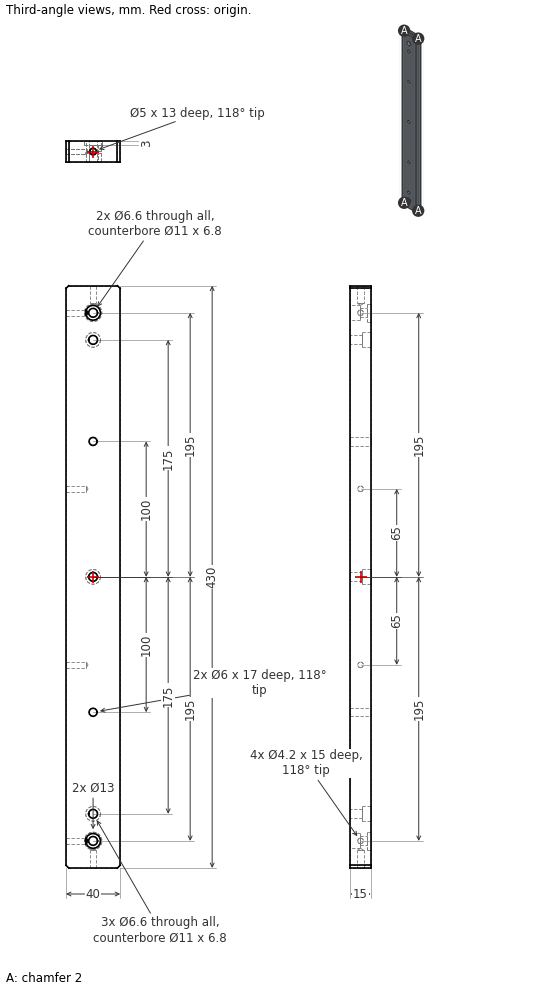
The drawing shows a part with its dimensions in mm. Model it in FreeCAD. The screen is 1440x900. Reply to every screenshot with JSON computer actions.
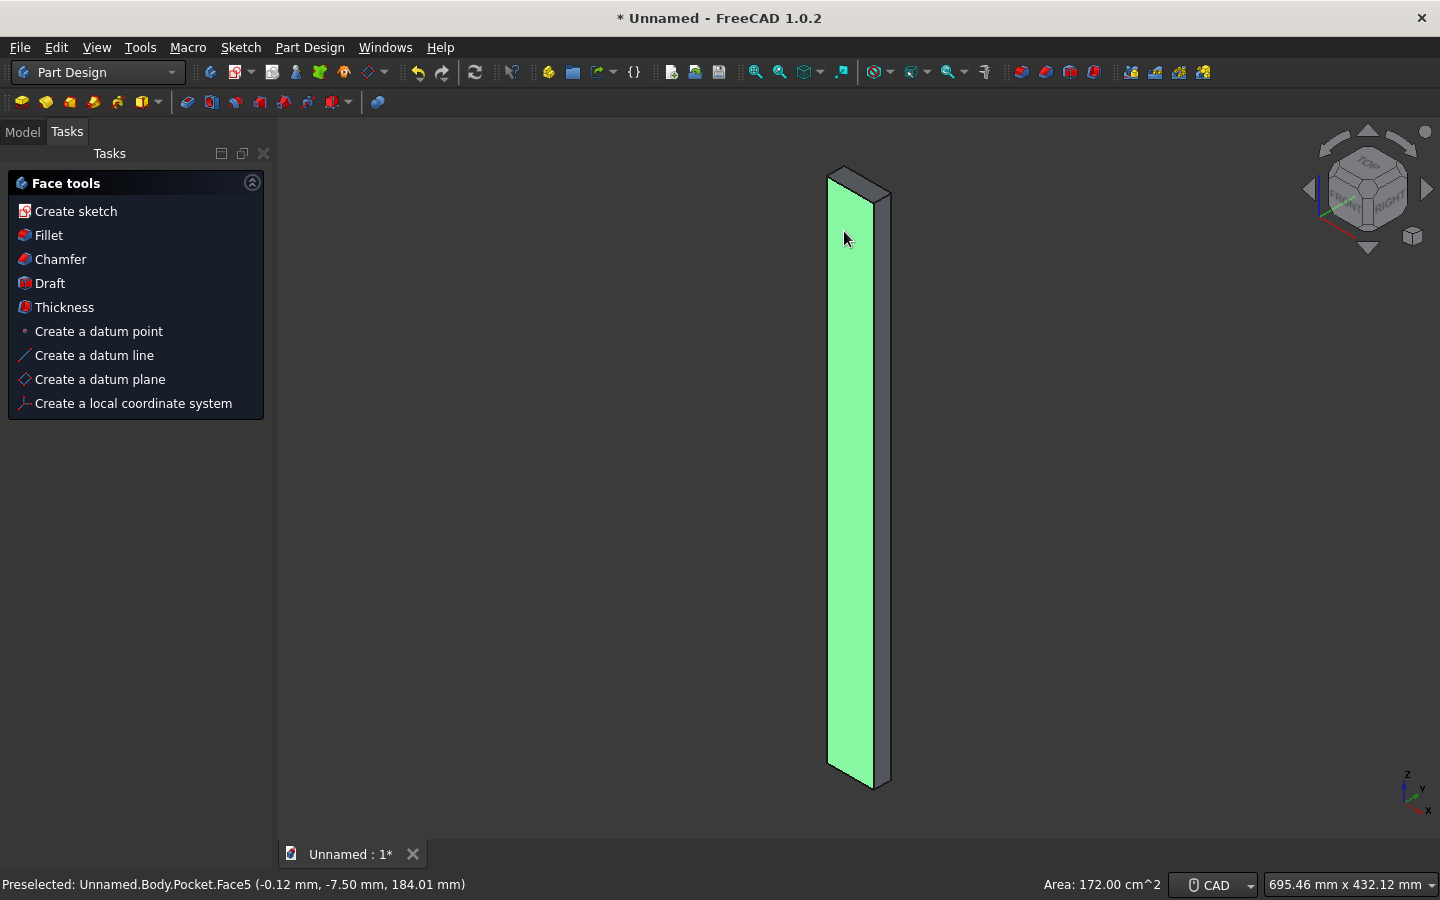
{"action": "left_click", "coordinate": [236, 72]}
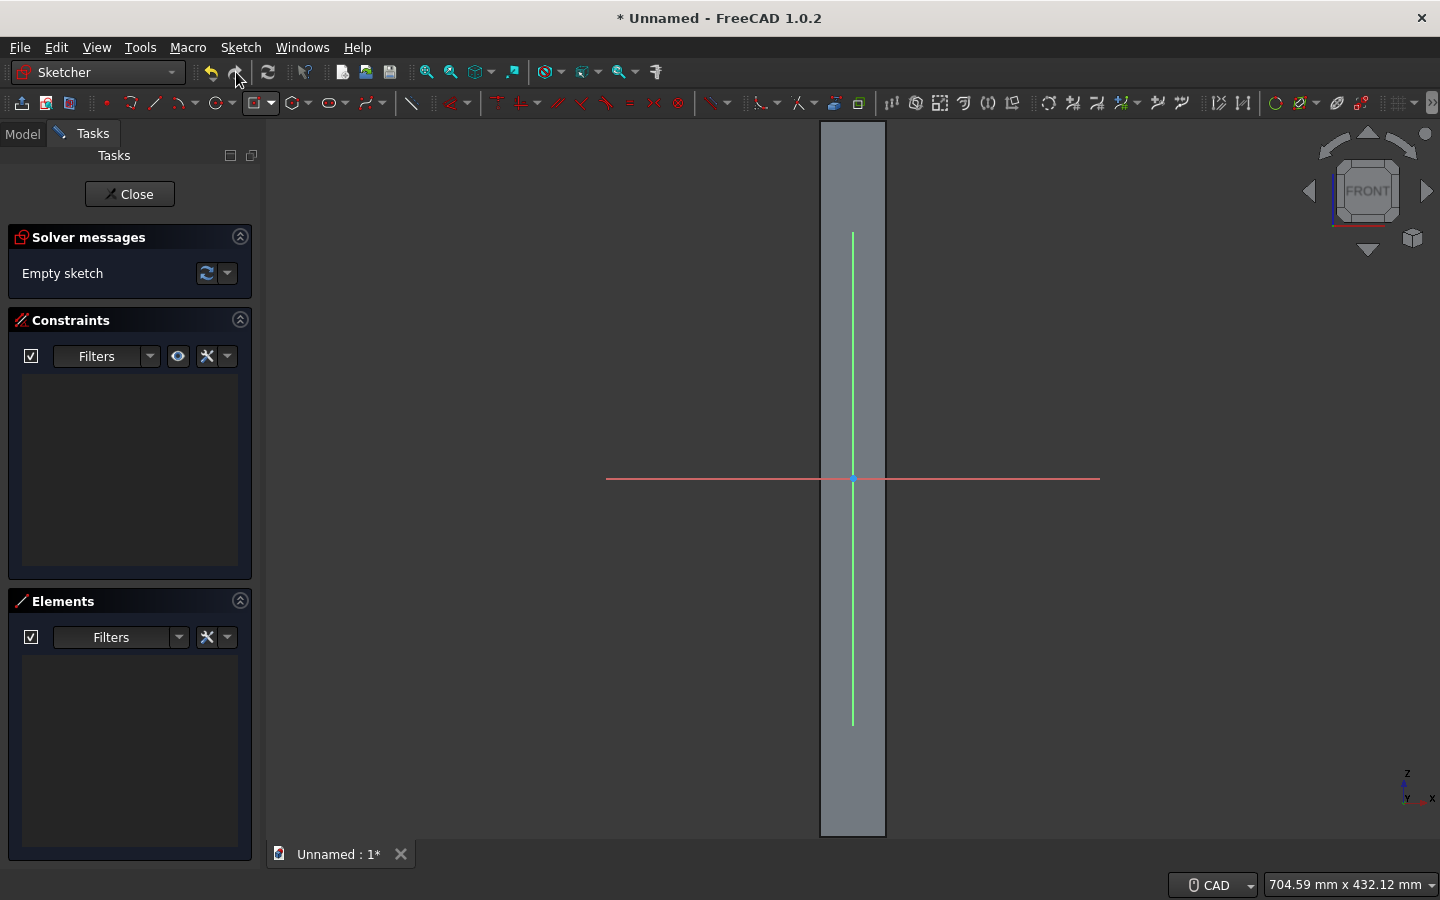
{"action": "scroll", "coordinate": [645, 479], "scroll_direction": "down", "scroll_amount": 2}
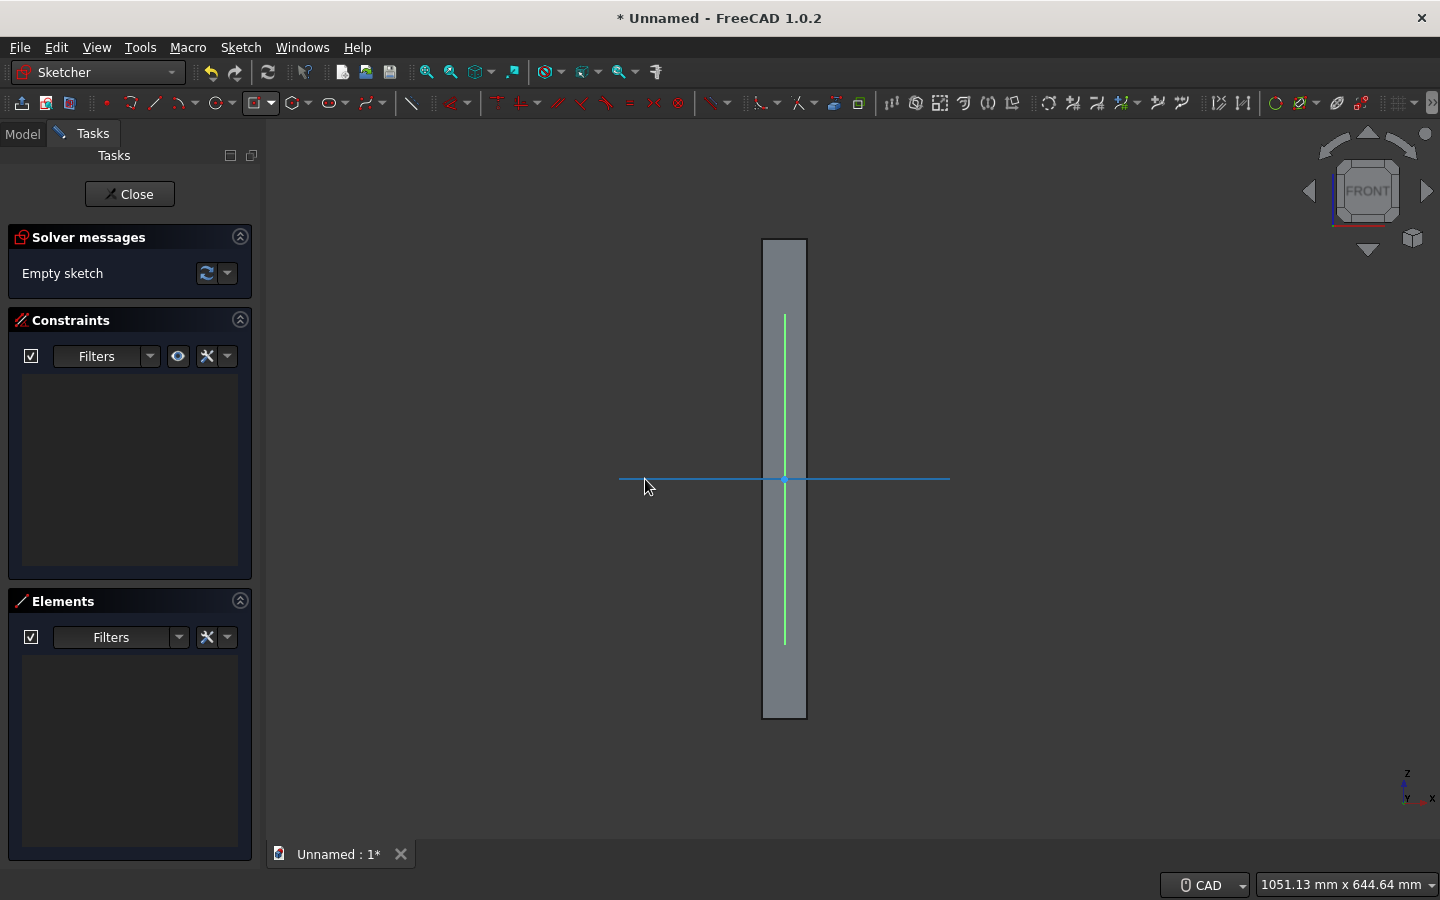
{"action": "key", "text": "g c"}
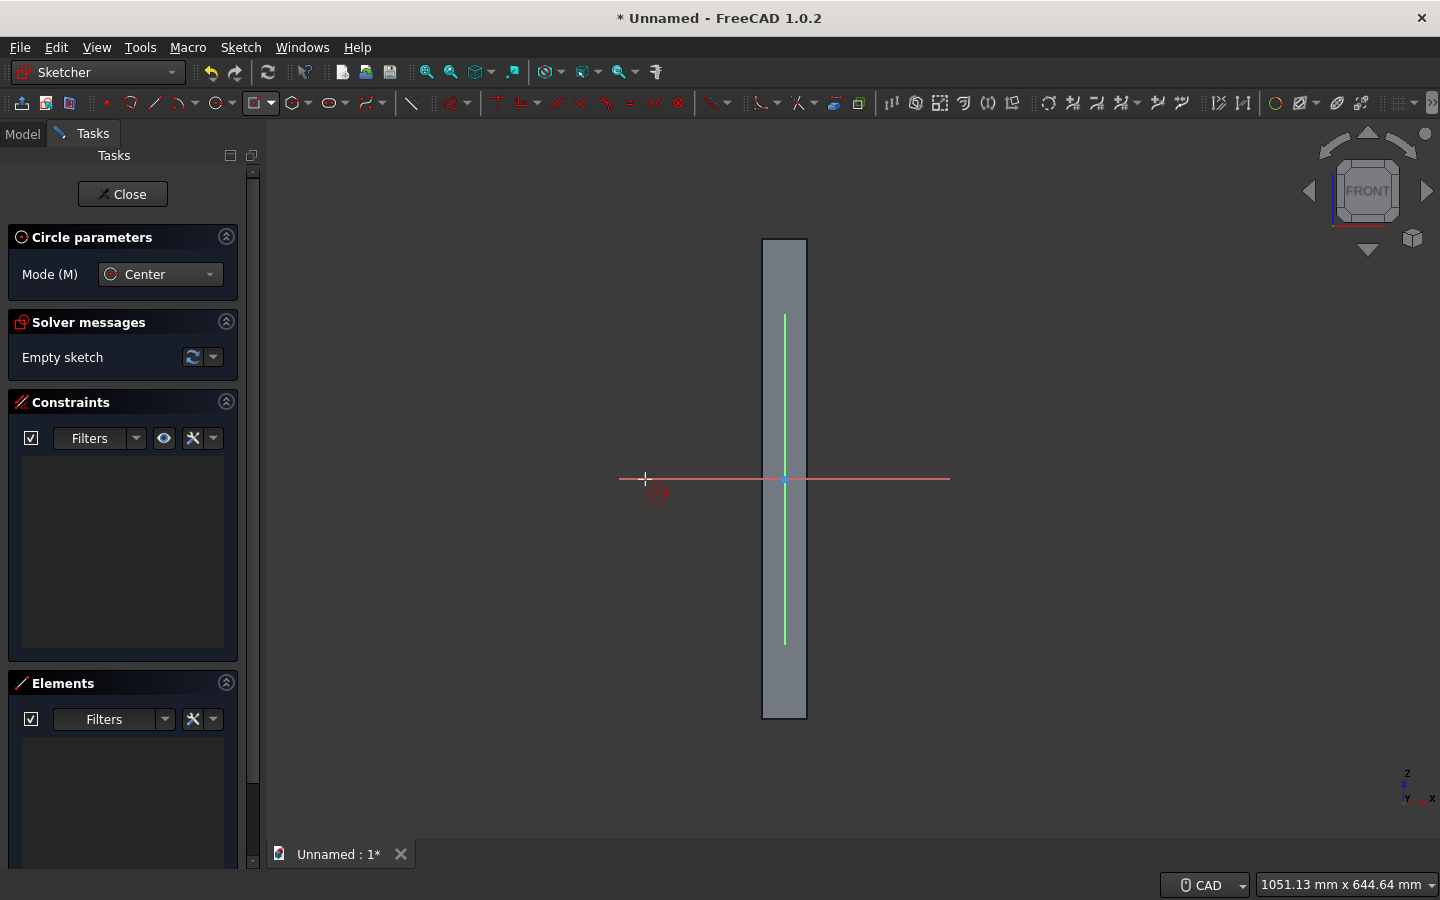
{"action": "scroll", "coordinate": [785, 261], "scroll_direction": "up", "scroll_amount": 10}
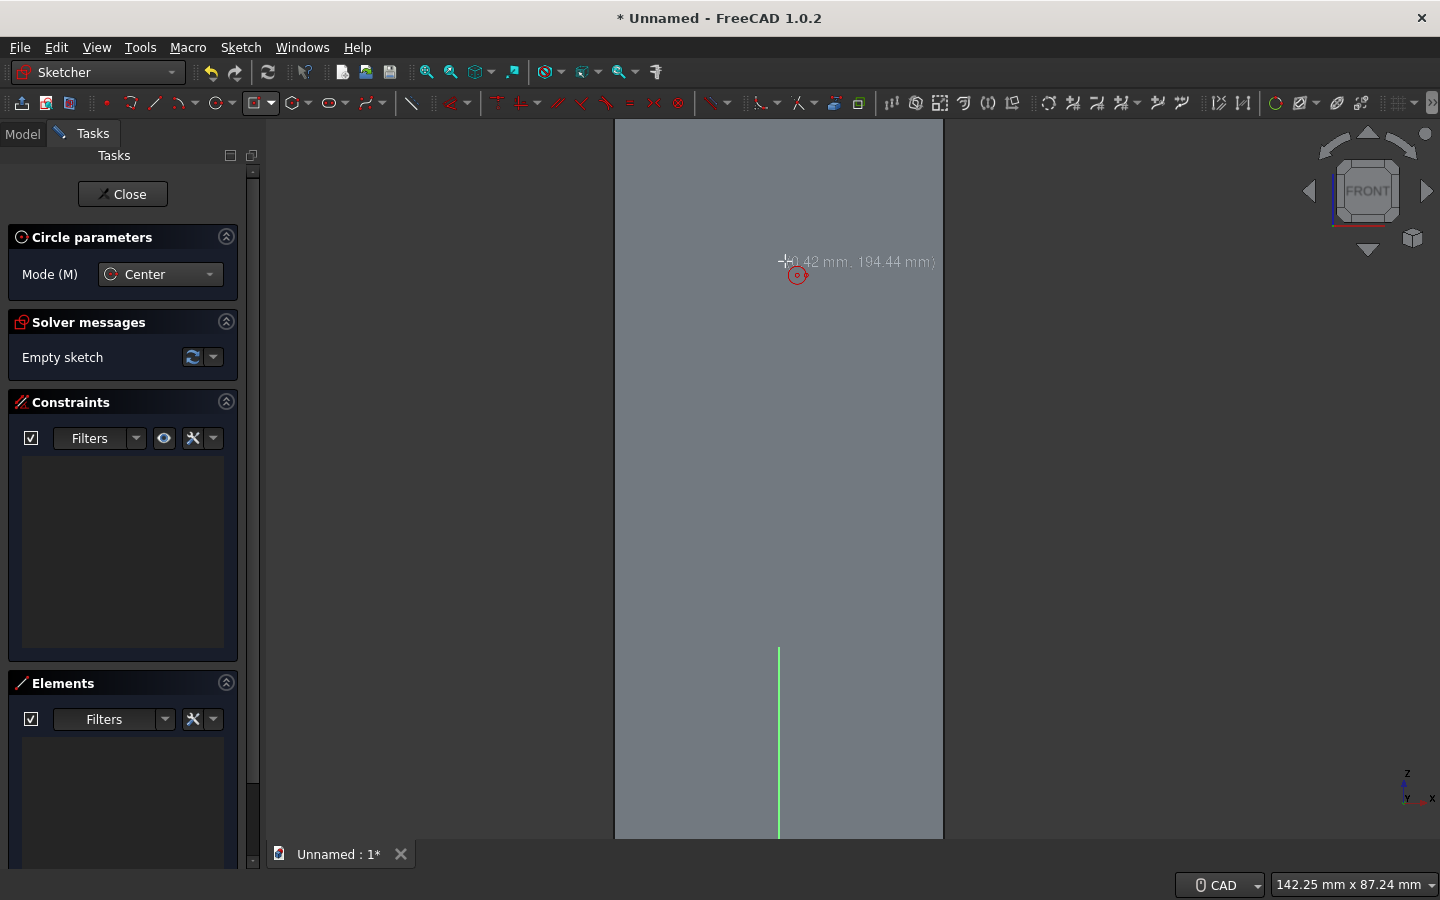
{"action": "scroll", "coordinate": [785, 261], "scroll_direction": "down", "scroll_amount": 10}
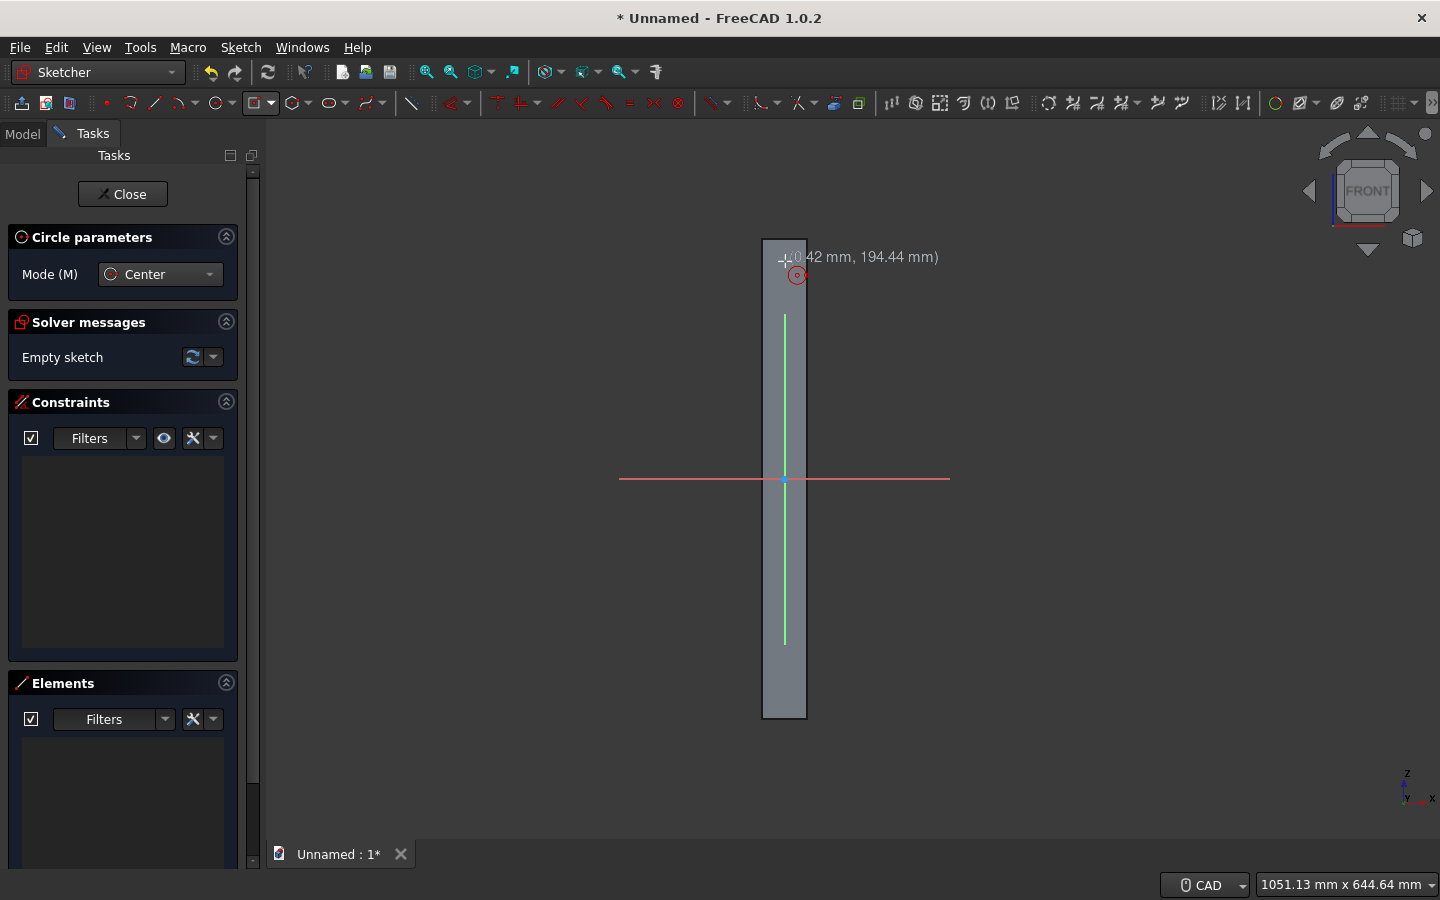
{"action": "left_click", "coordinate": [785, 261]}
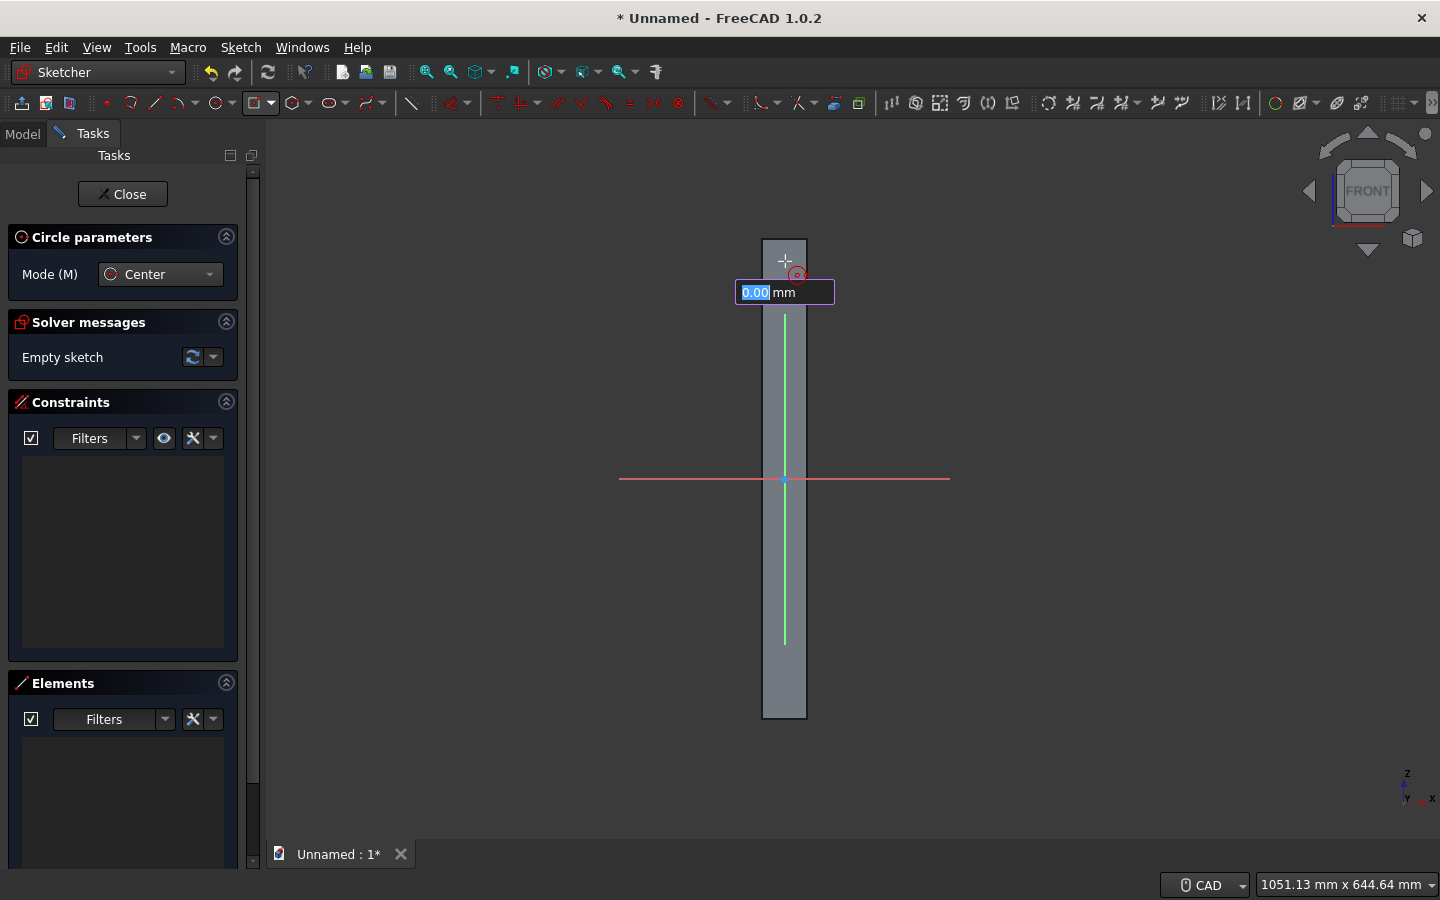
{"action": "scroll", "coordinate": [788, 260], "scroll_direction": "up", "scroll_amount": 8}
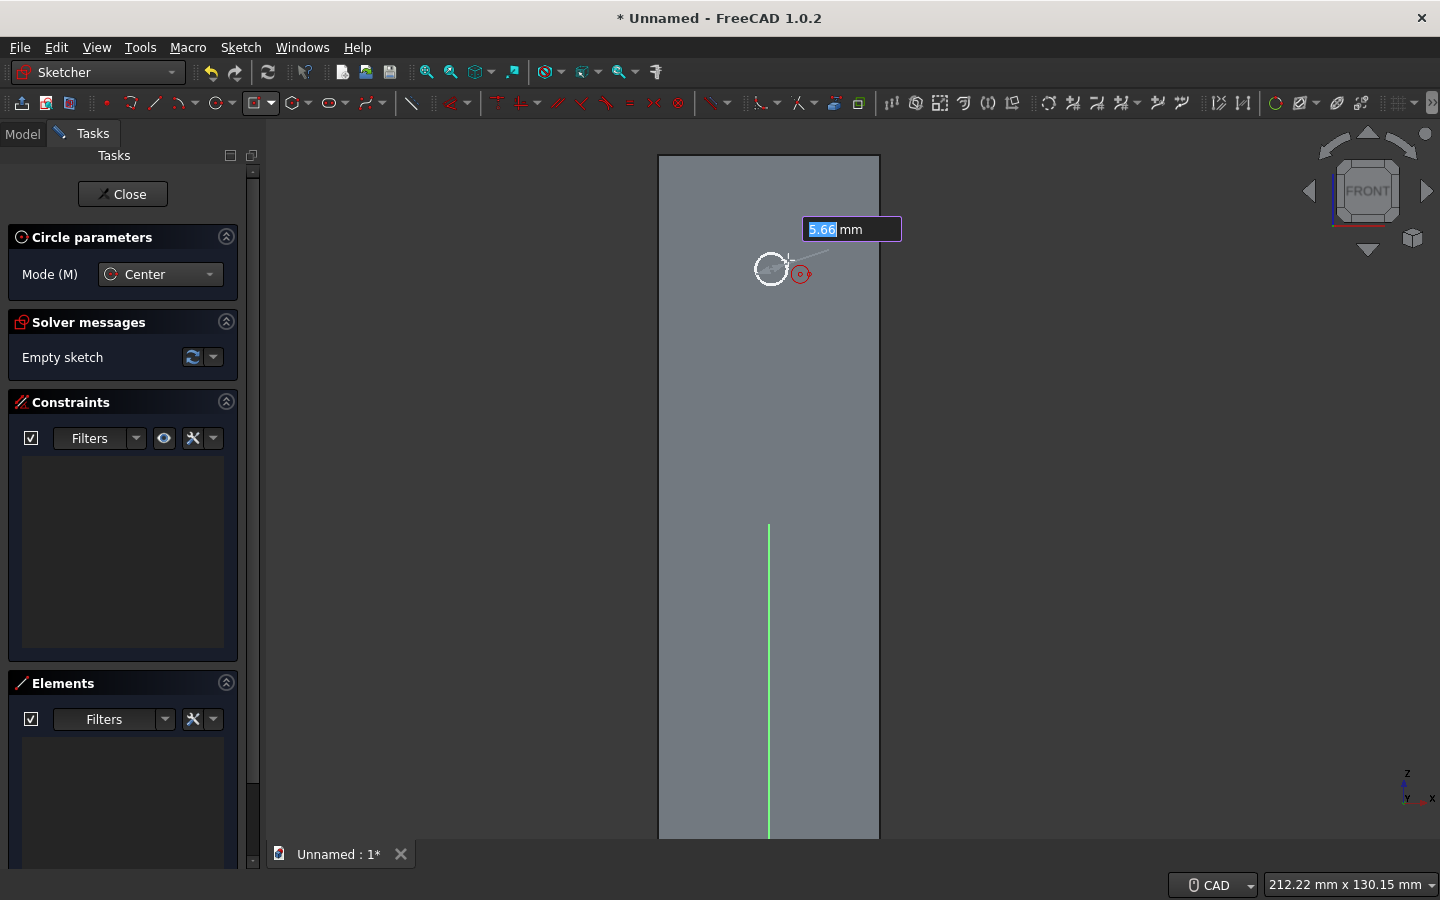
{"action": "left_click", "coordinate": [786, 260]}